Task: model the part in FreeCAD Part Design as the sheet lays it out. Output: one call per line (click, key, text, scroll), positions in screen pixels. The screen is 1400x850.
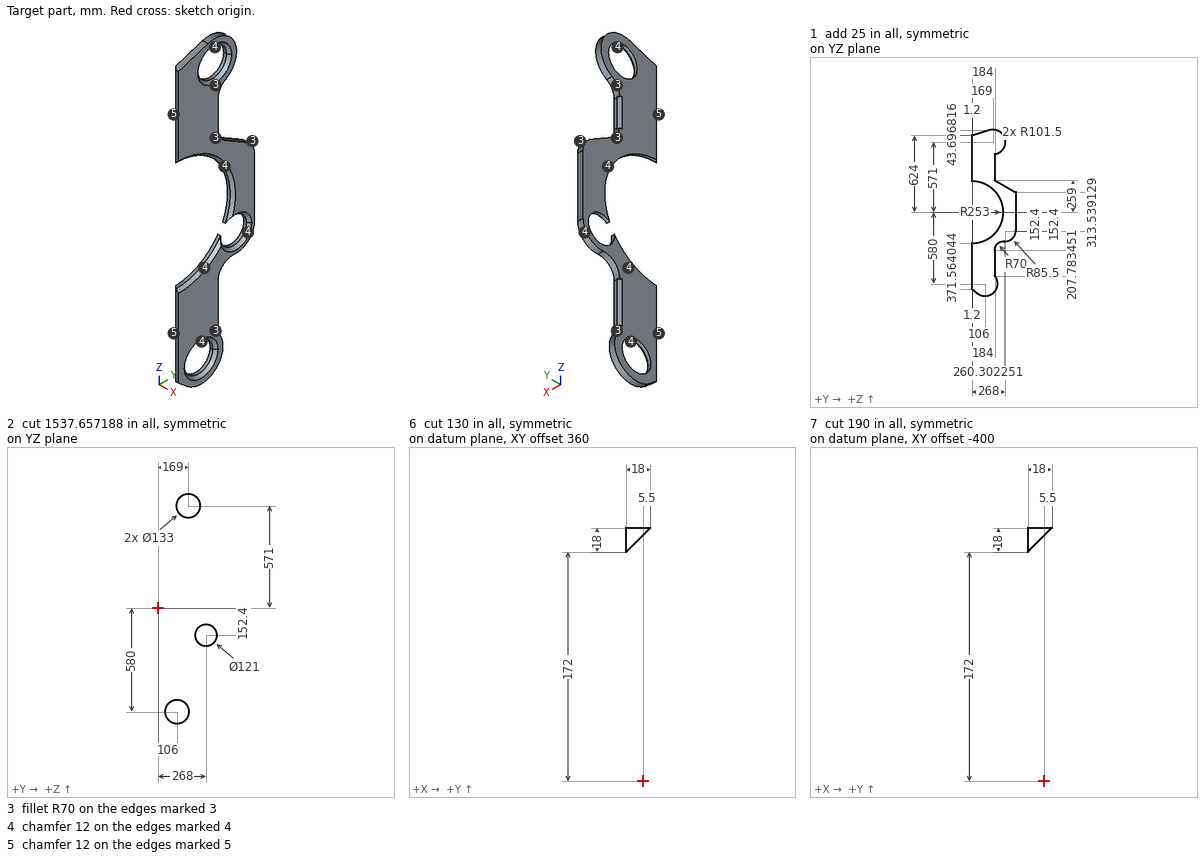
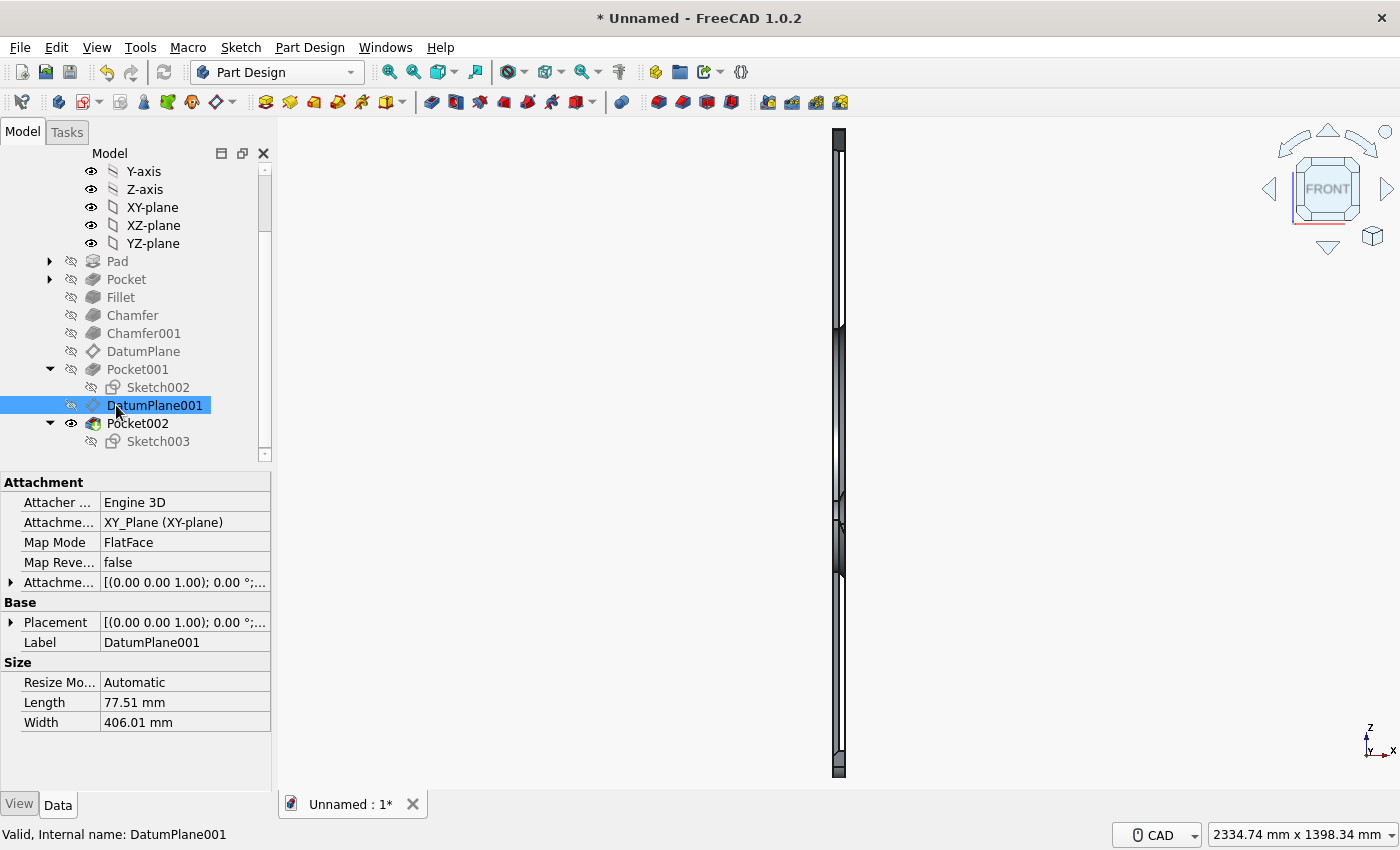
key(0)